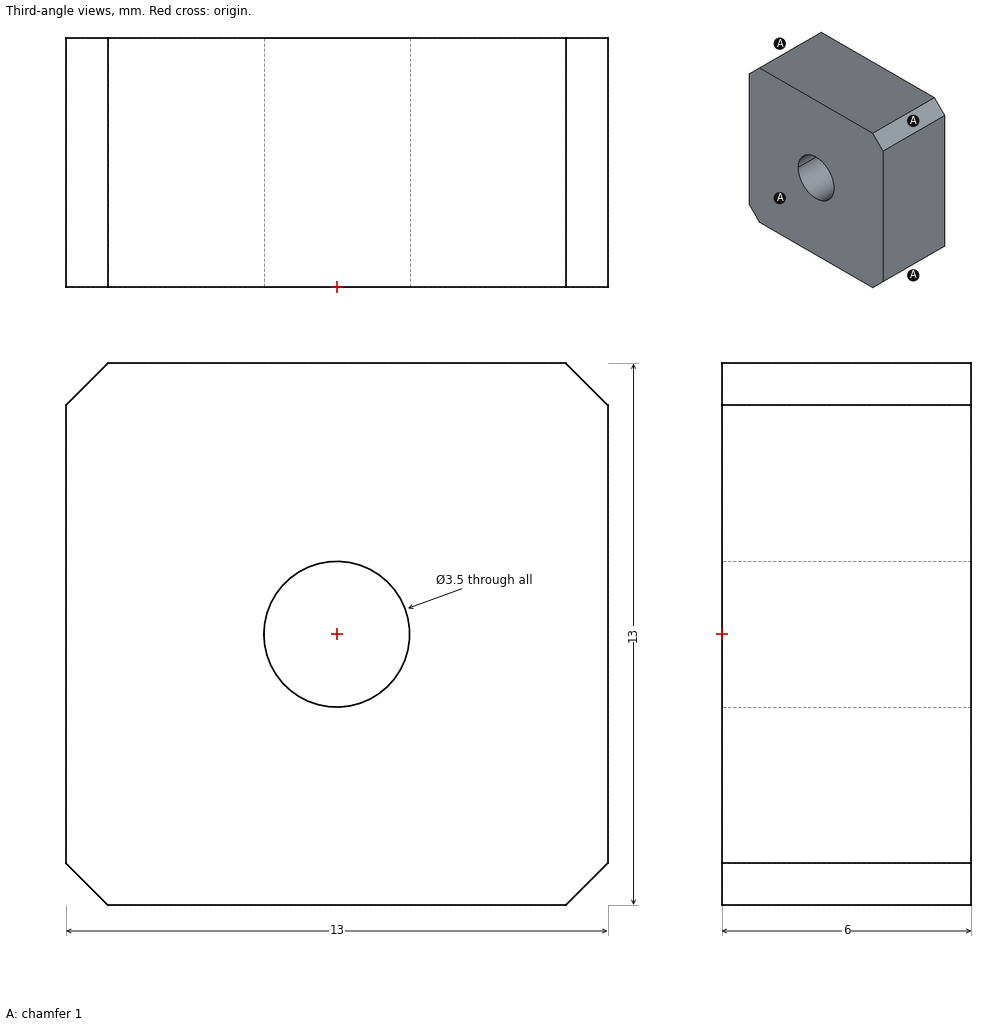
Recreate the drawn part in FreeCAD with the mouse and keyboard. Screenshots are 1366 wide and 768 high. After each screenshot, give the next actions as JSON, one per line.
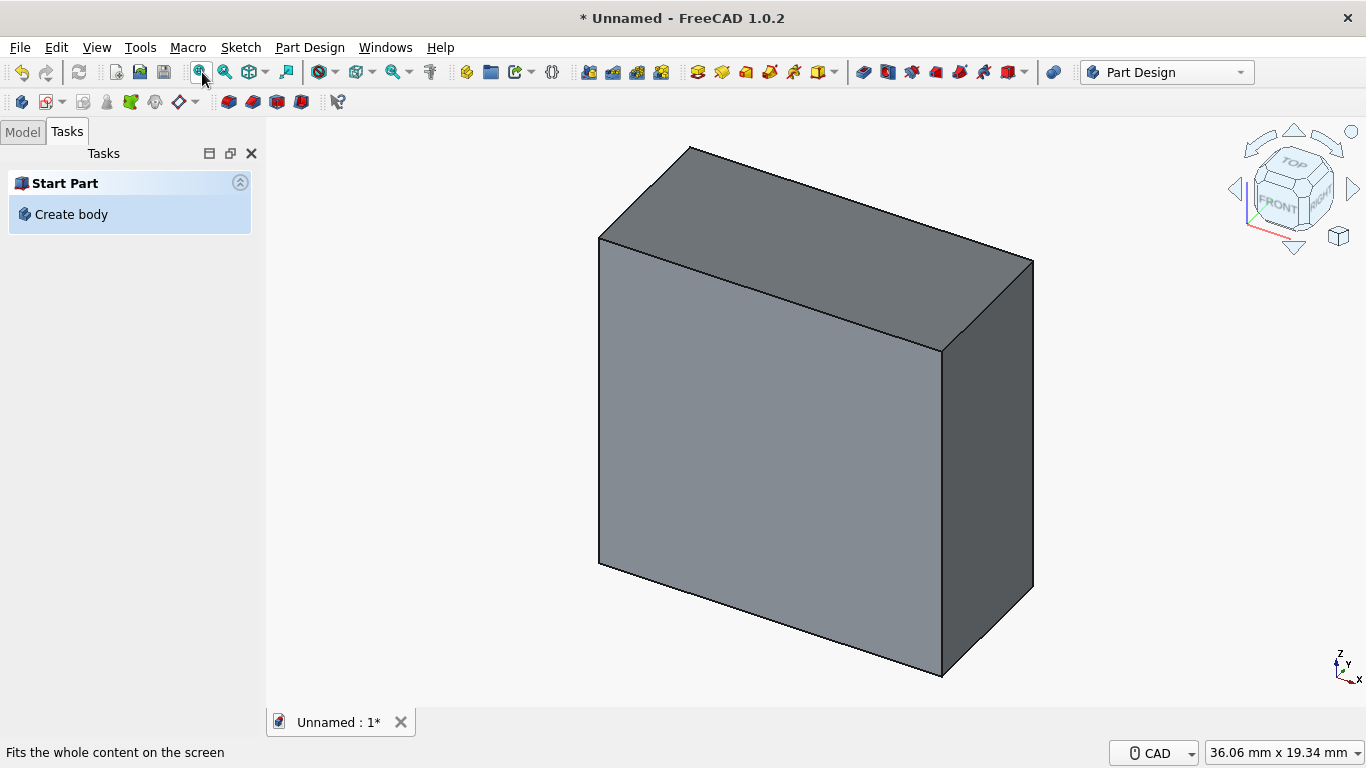
{"action": "key", "text": "4"}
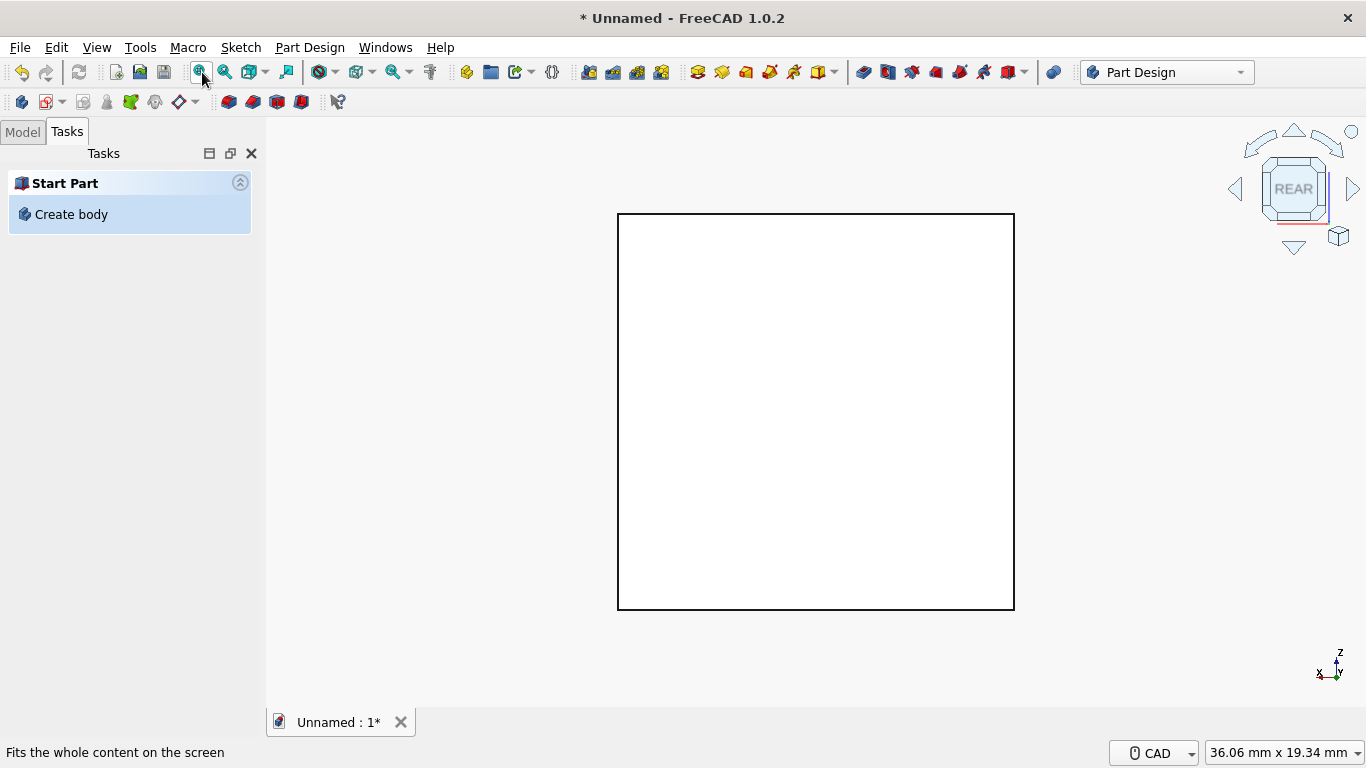
{"action": "left_click", "coordinate": [816, 411]}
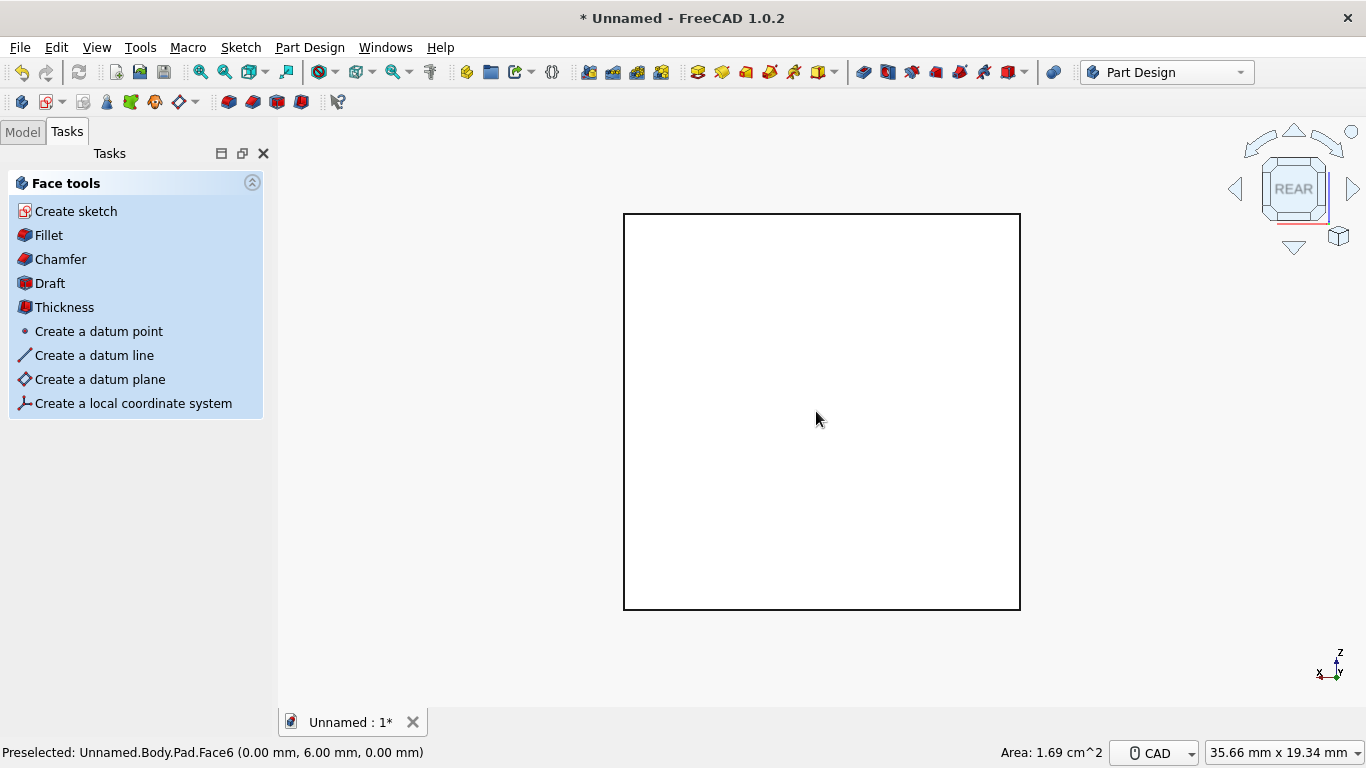
{"action": "left_click", "coordinate": [46, 102]}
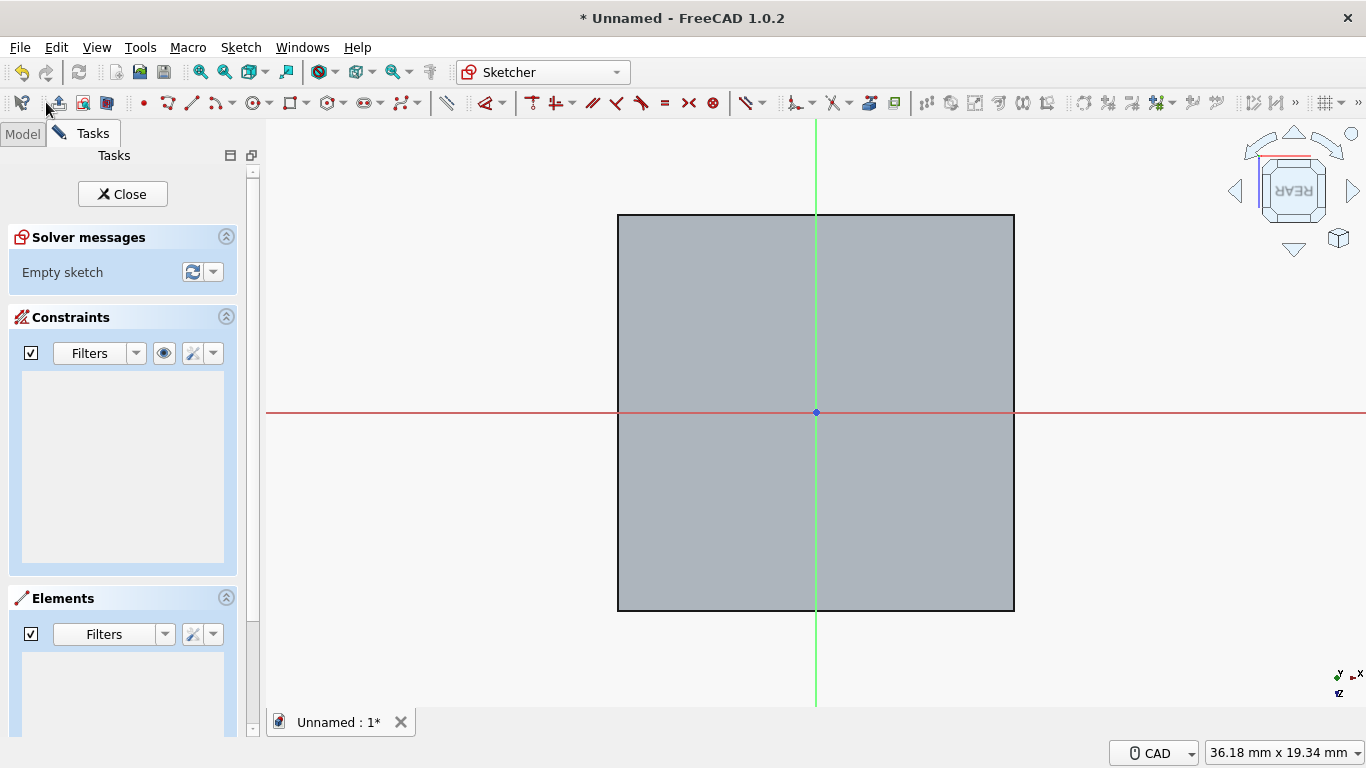
{"action": "scroll", "coordinate": [846, 413], "scroll_direction": "up", "scroll_amount": 6}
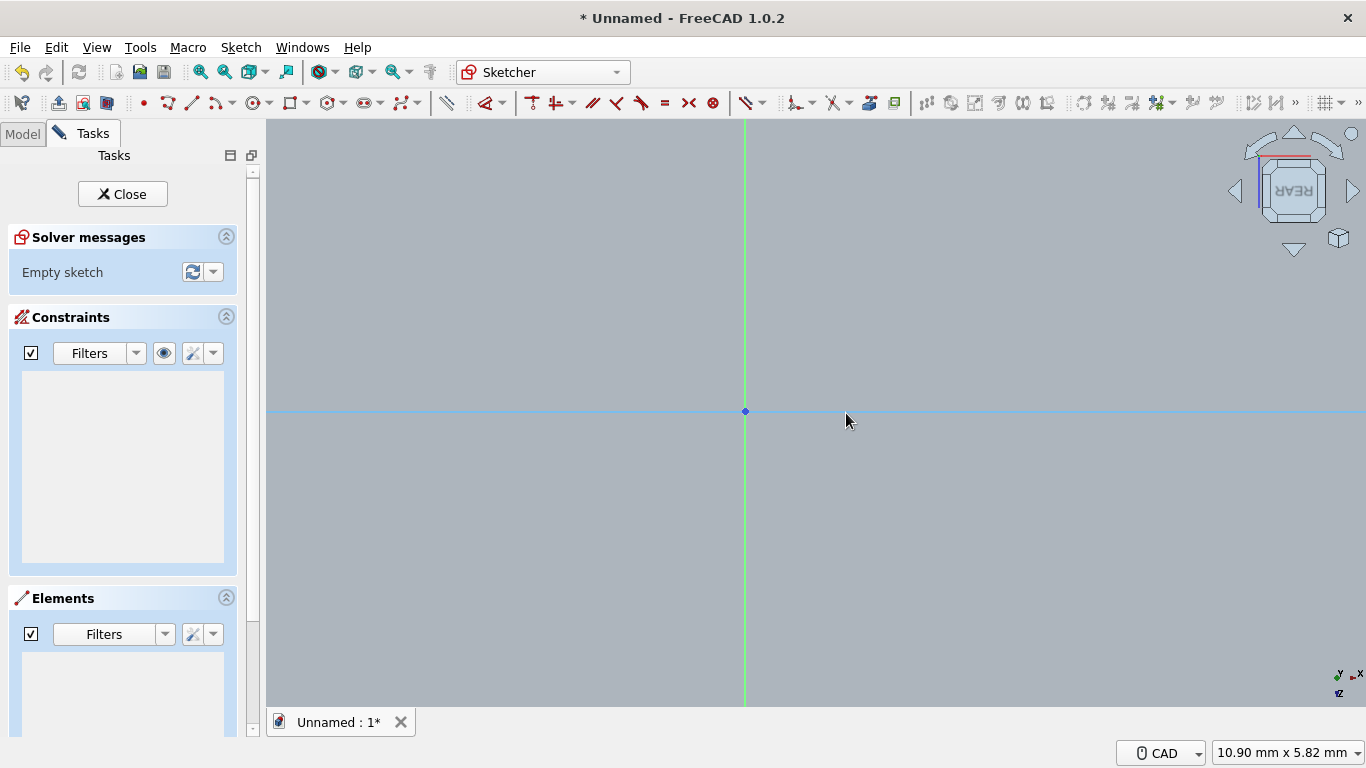
{"action": "left_click", "coordinate": [254, 104]}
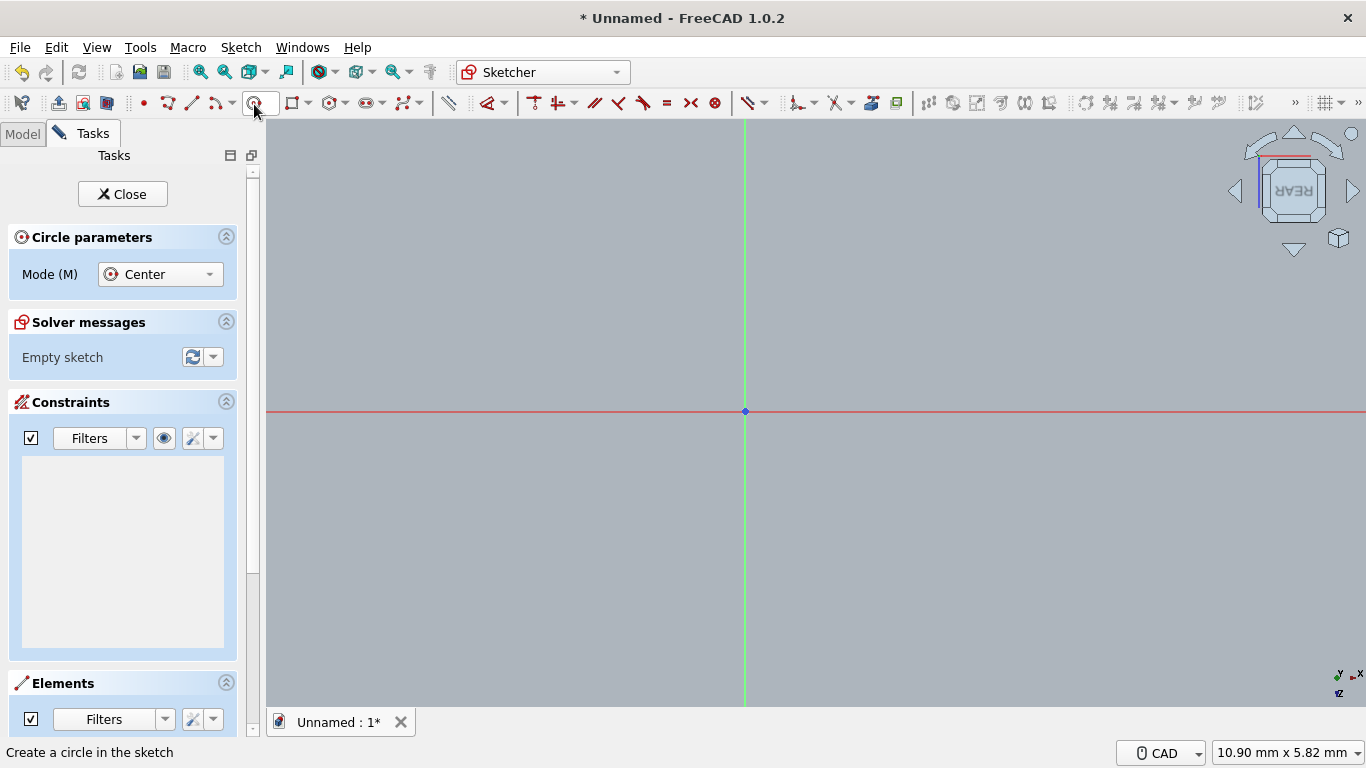
{"action": "left_click", "coordinate": [745, 412]}
{"action": "left_click", "coordinate": [870, 287]}
{"action": "key", "text": "Escape"}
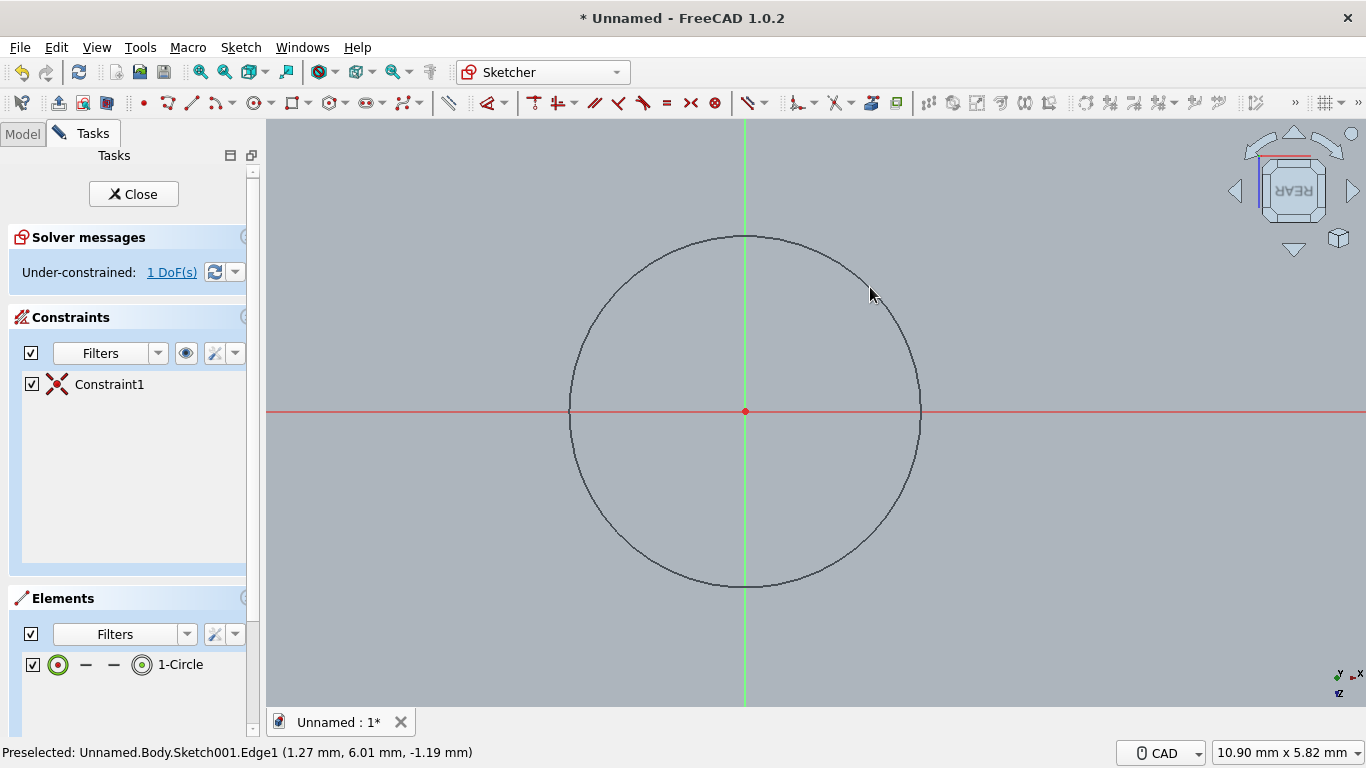
{"action": "key", "text": "d"}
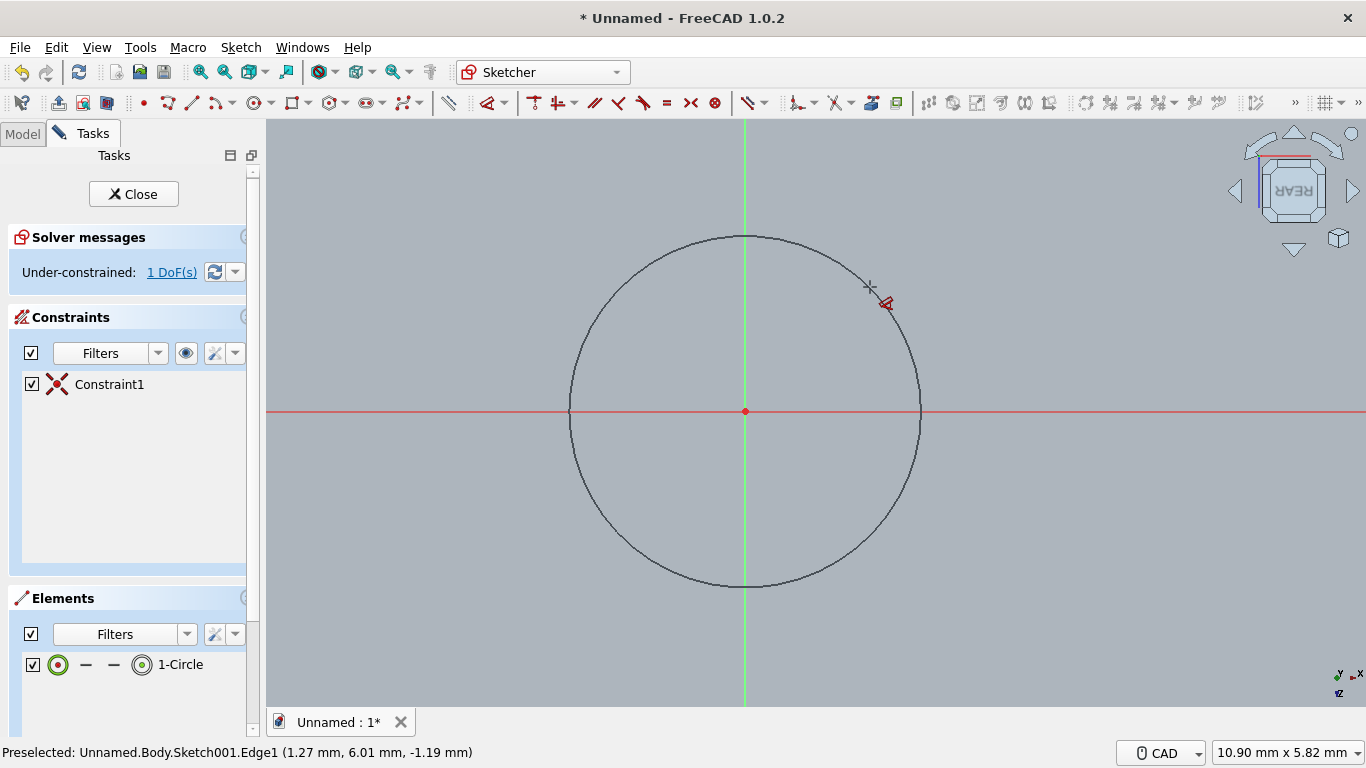
{"action": "left_click", "coordinate": [869, 287]}
{"action": "left_click", "coordinate": [892, 264]}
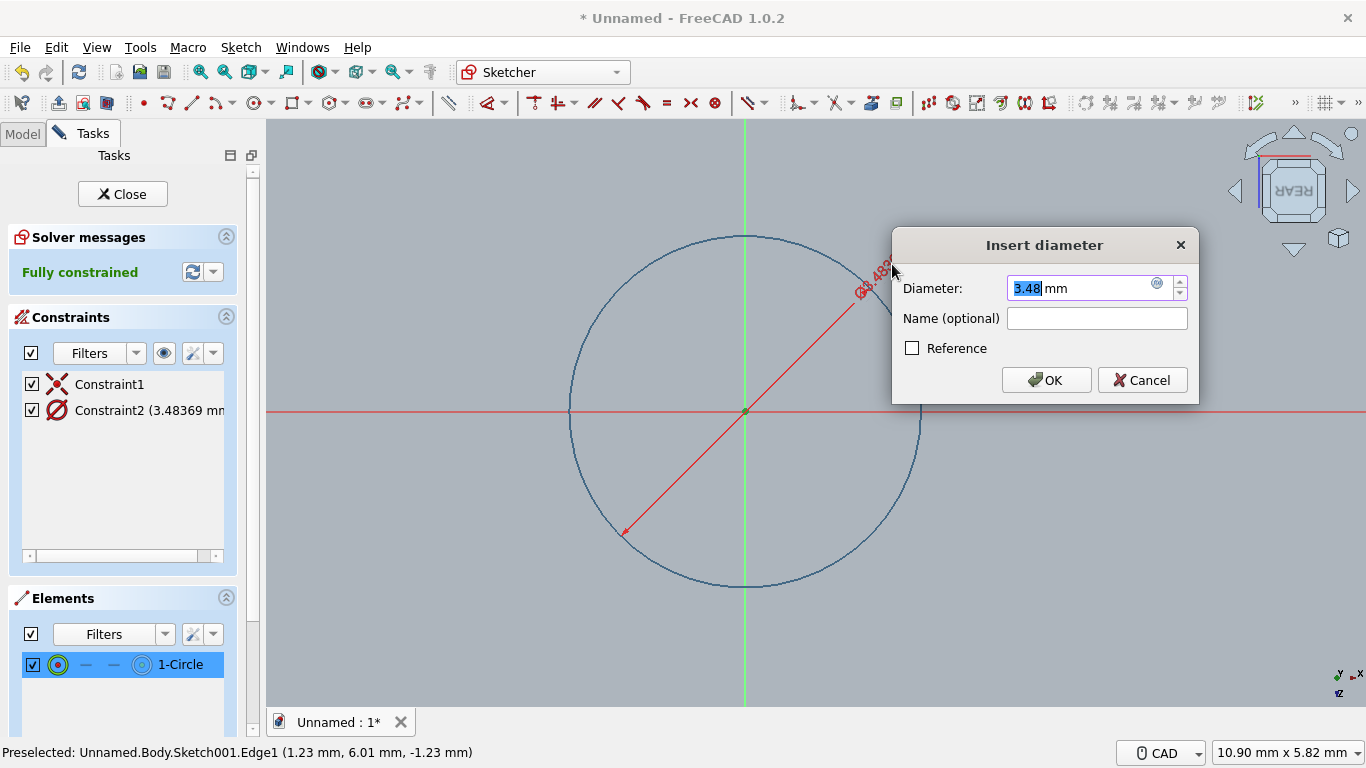
{"action": "type", "text": "3.5"}
{"action": "key", "text": "Return"}
{"action": "key", "text": "Escape"}